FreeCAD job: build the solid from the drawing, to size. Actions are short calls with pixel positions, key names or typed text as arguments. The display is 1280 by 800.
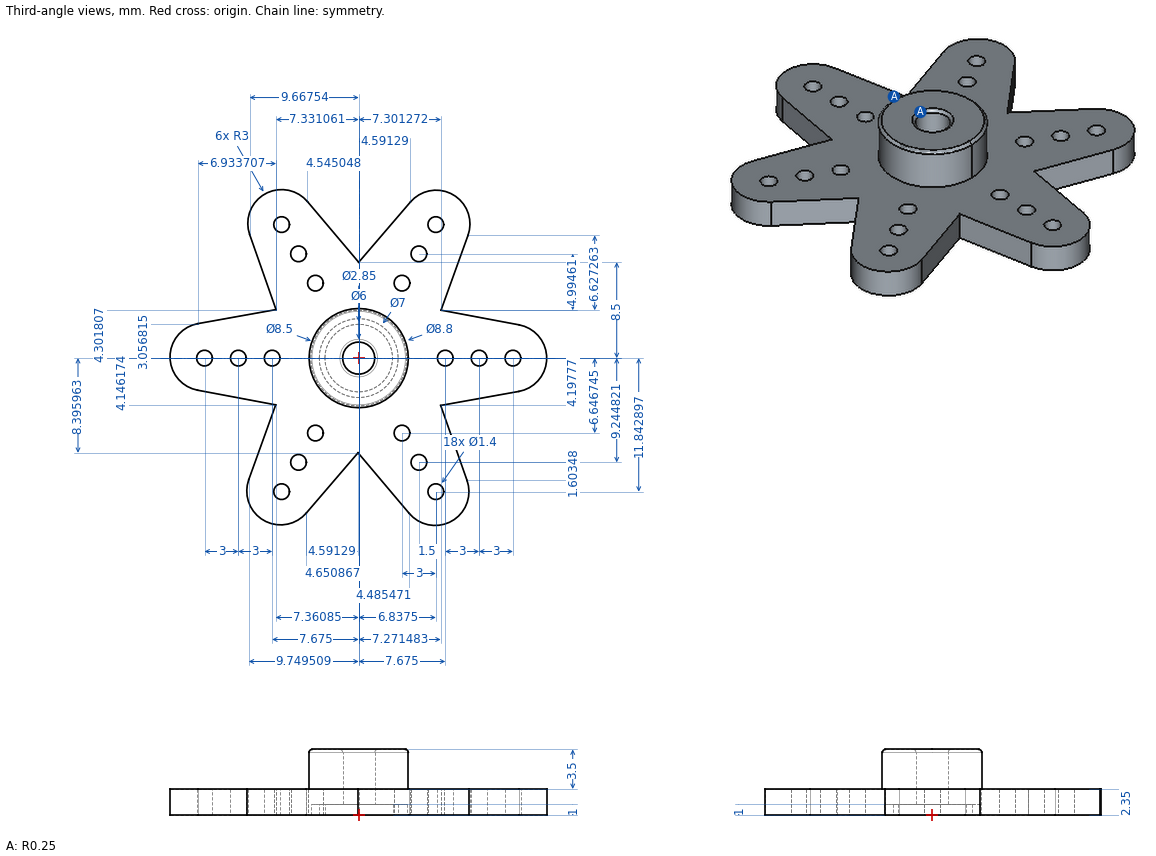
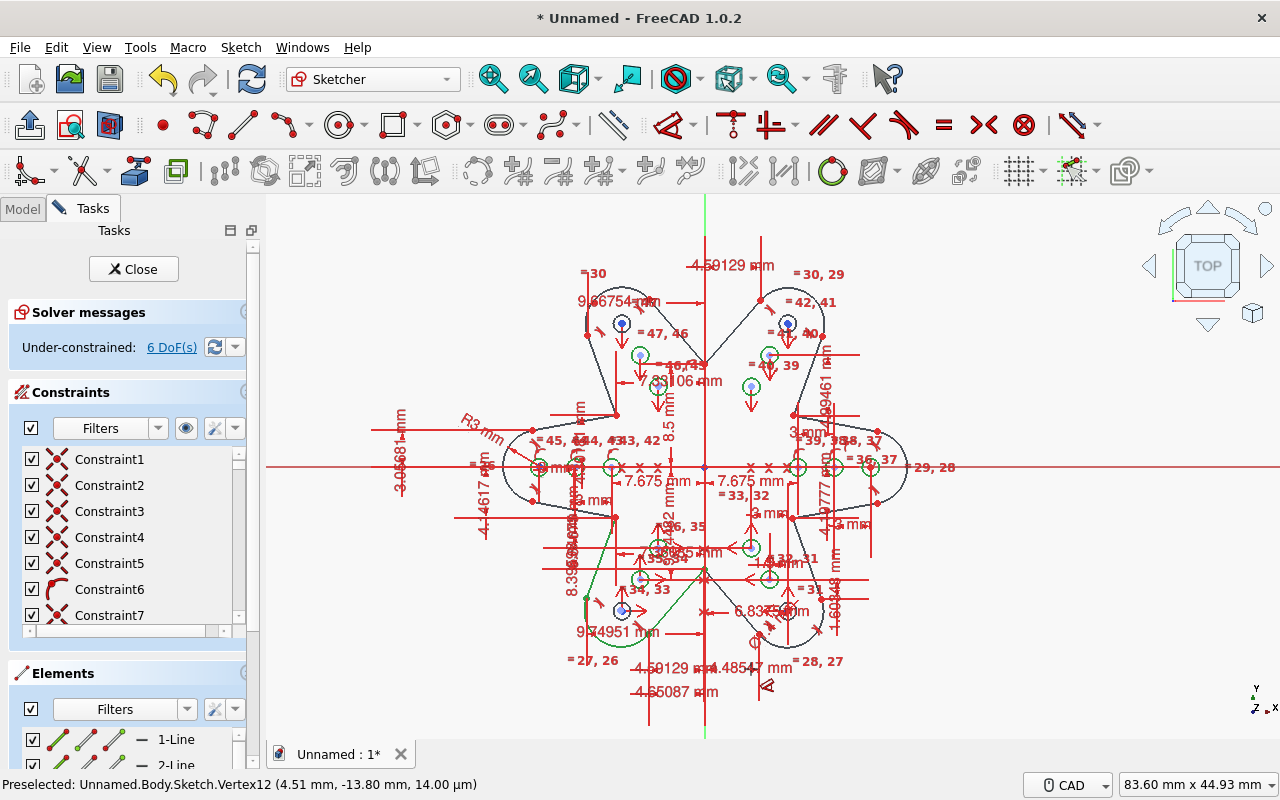
click(793, 518)
click(749, 409)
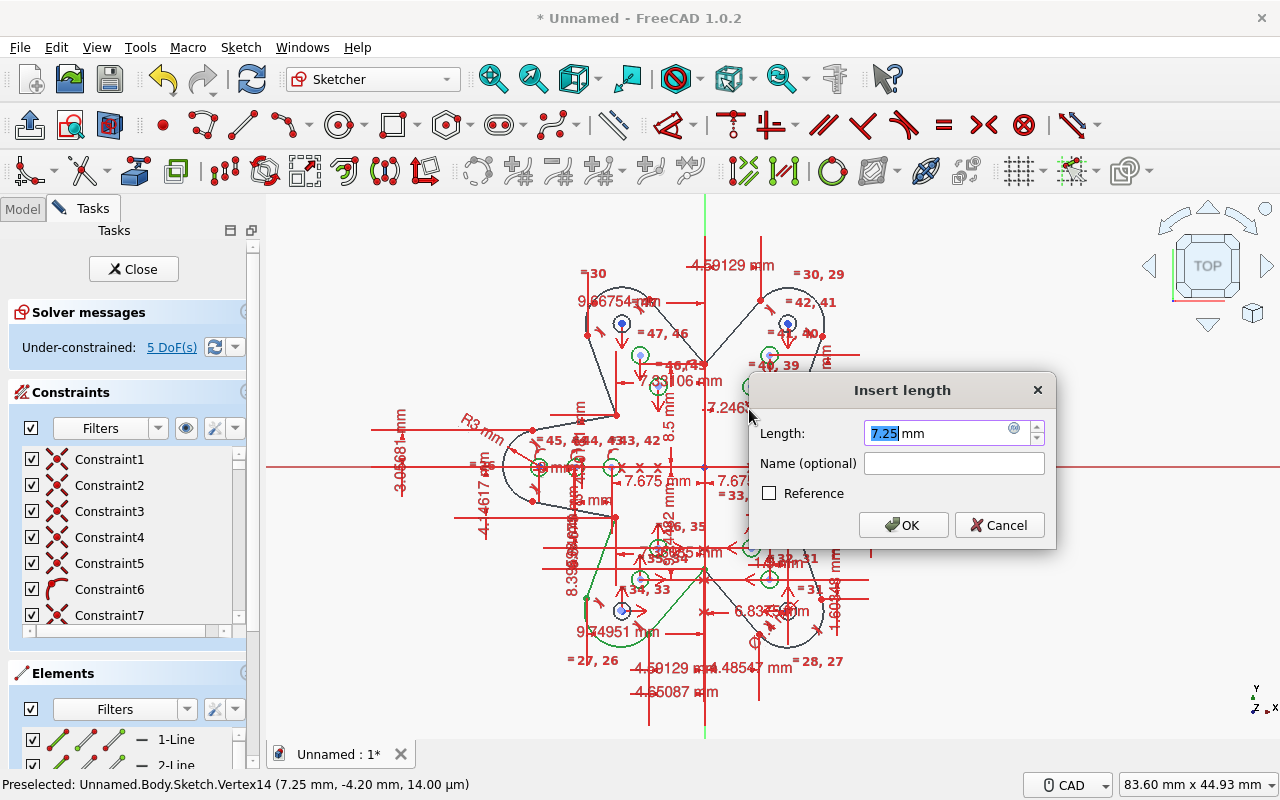
text(7.271483)
key(Return)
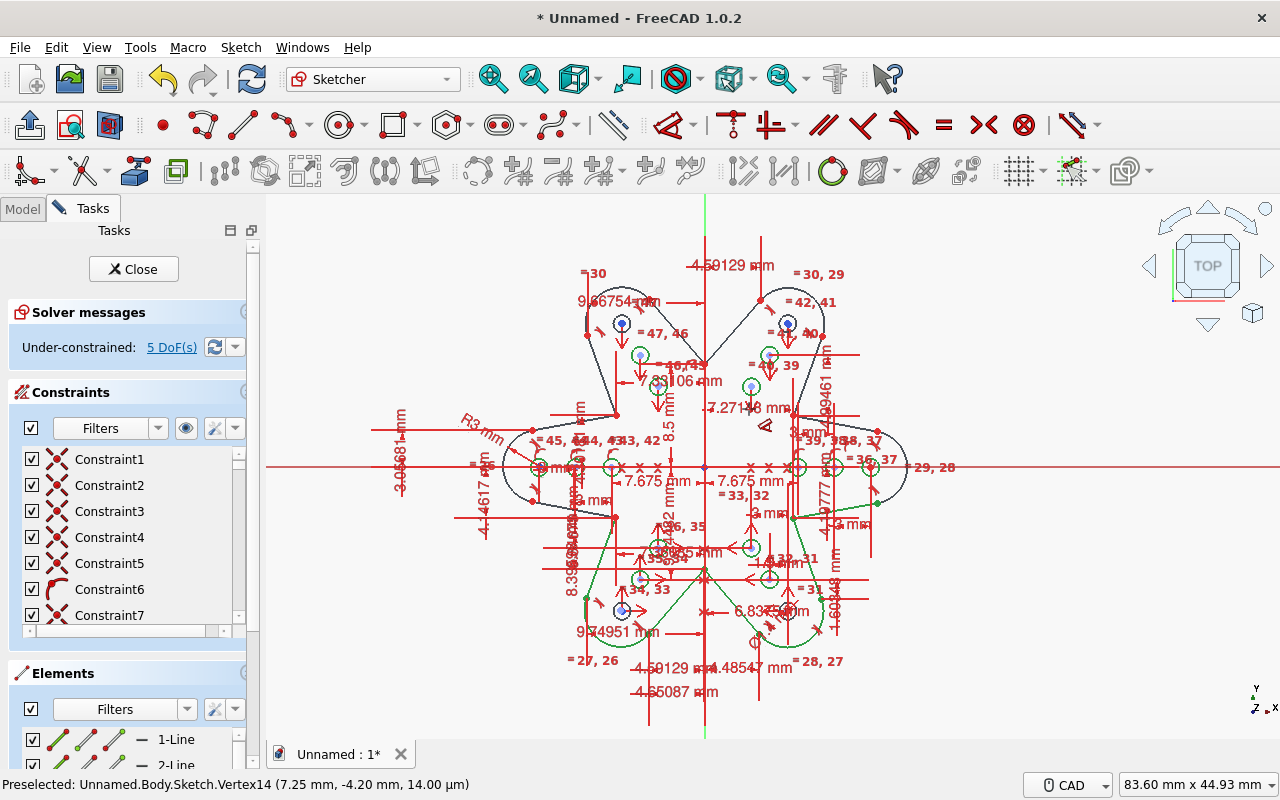
click(794, 416)
click(729, 358)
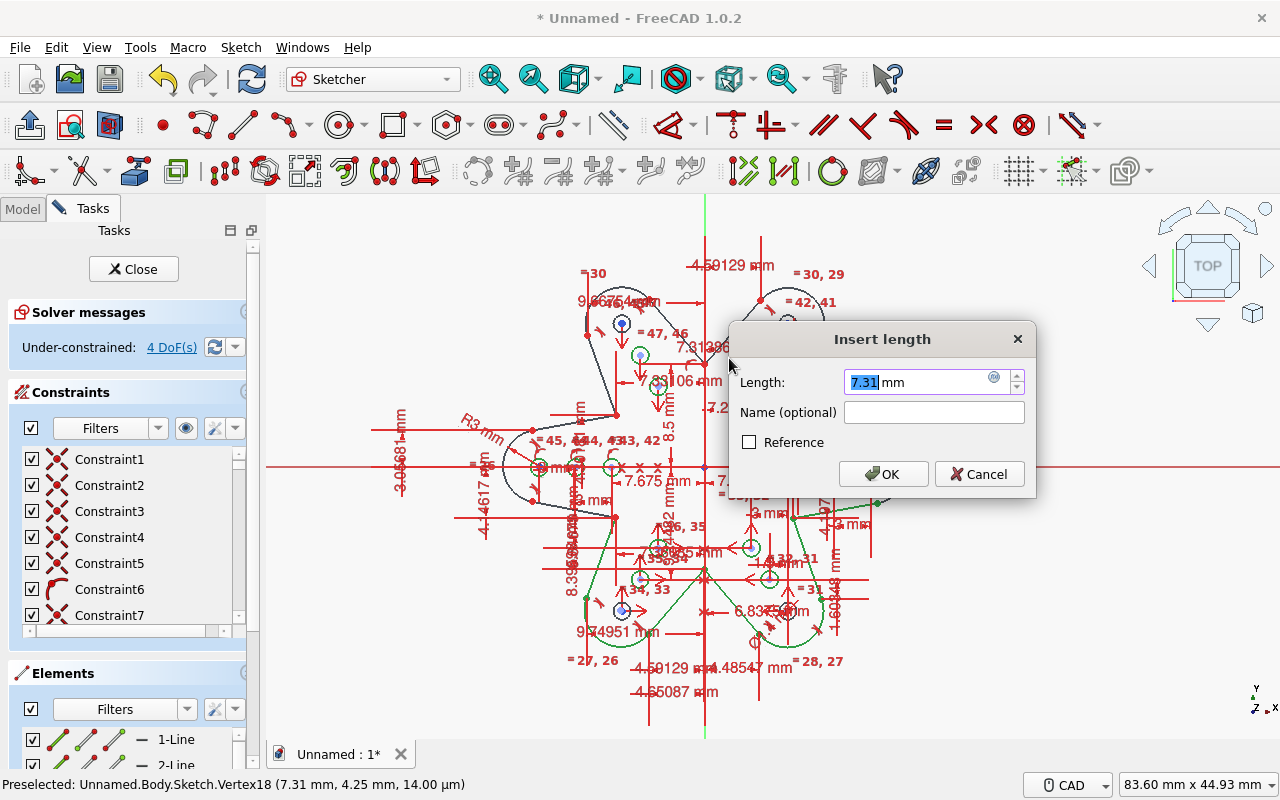
text(7.301272)
key(Return)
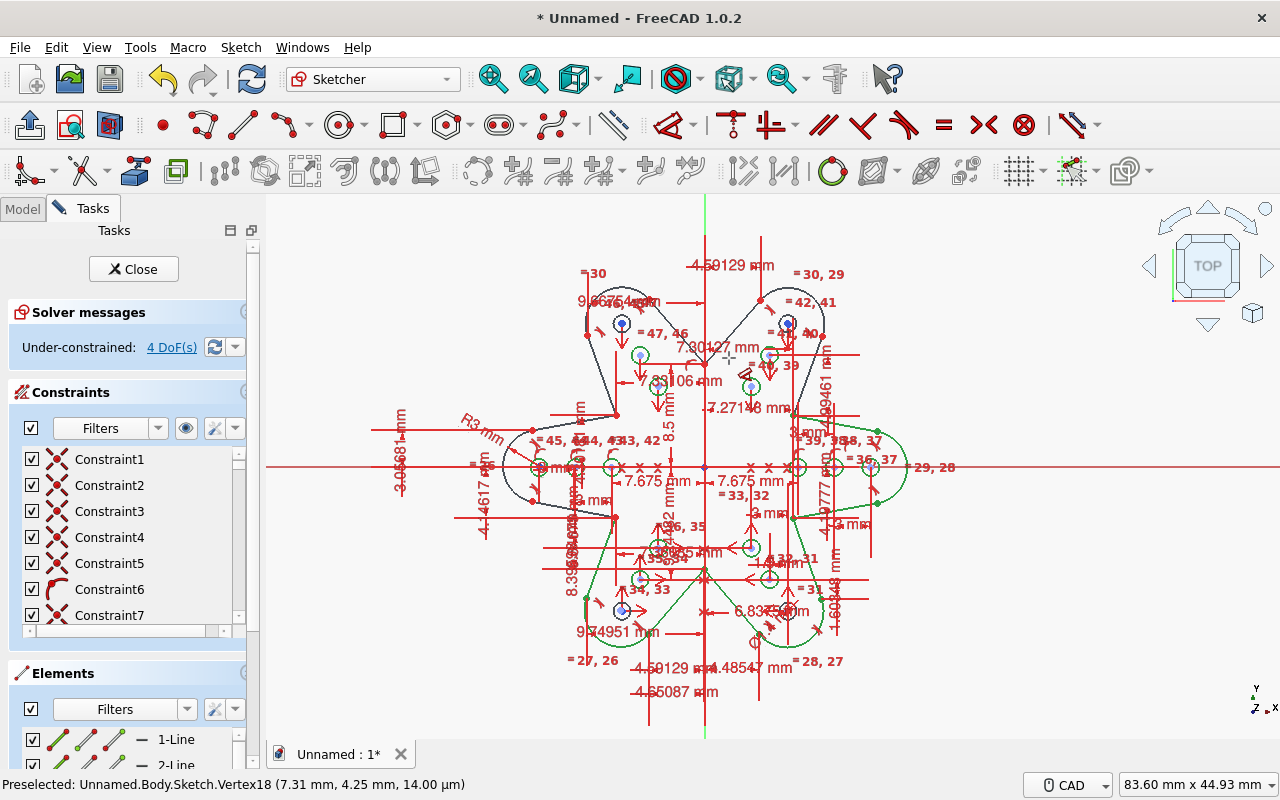
click(650, 300)
click(658, 266)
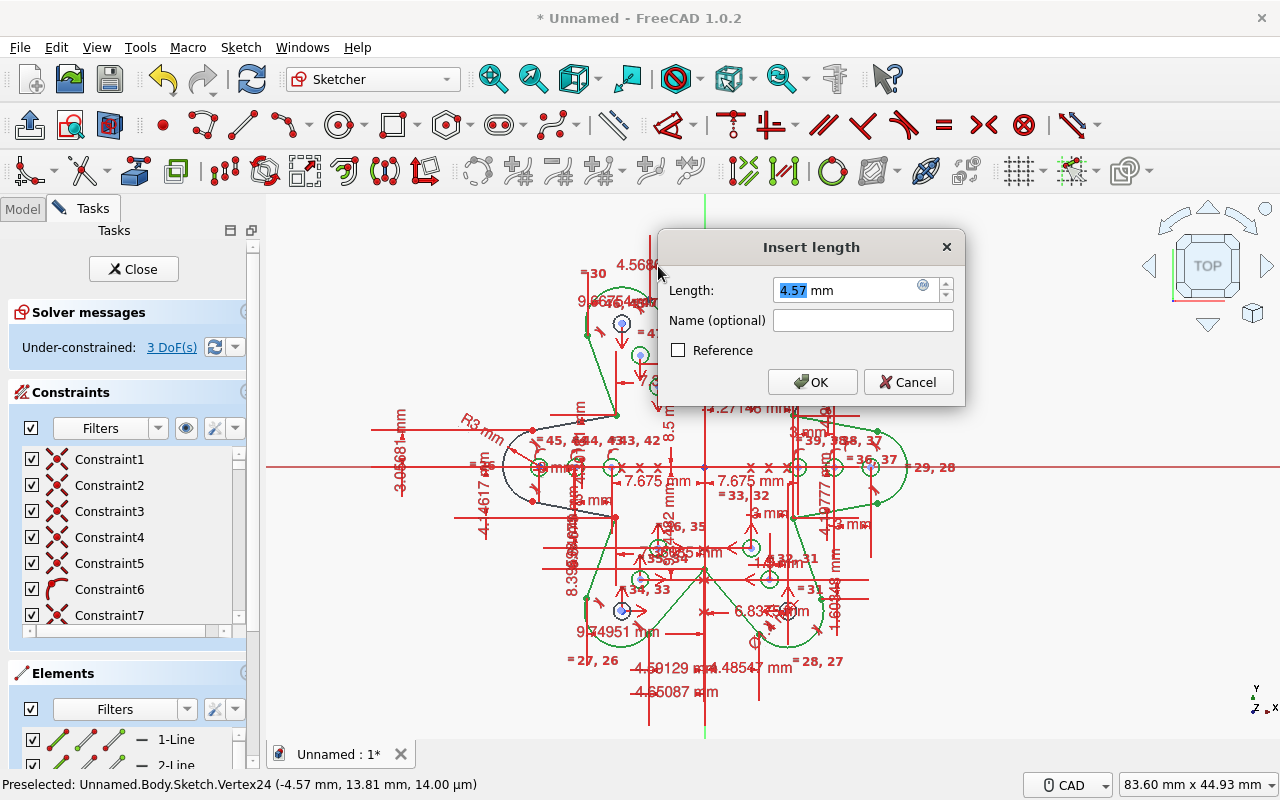
text(4.545048)
key(Return)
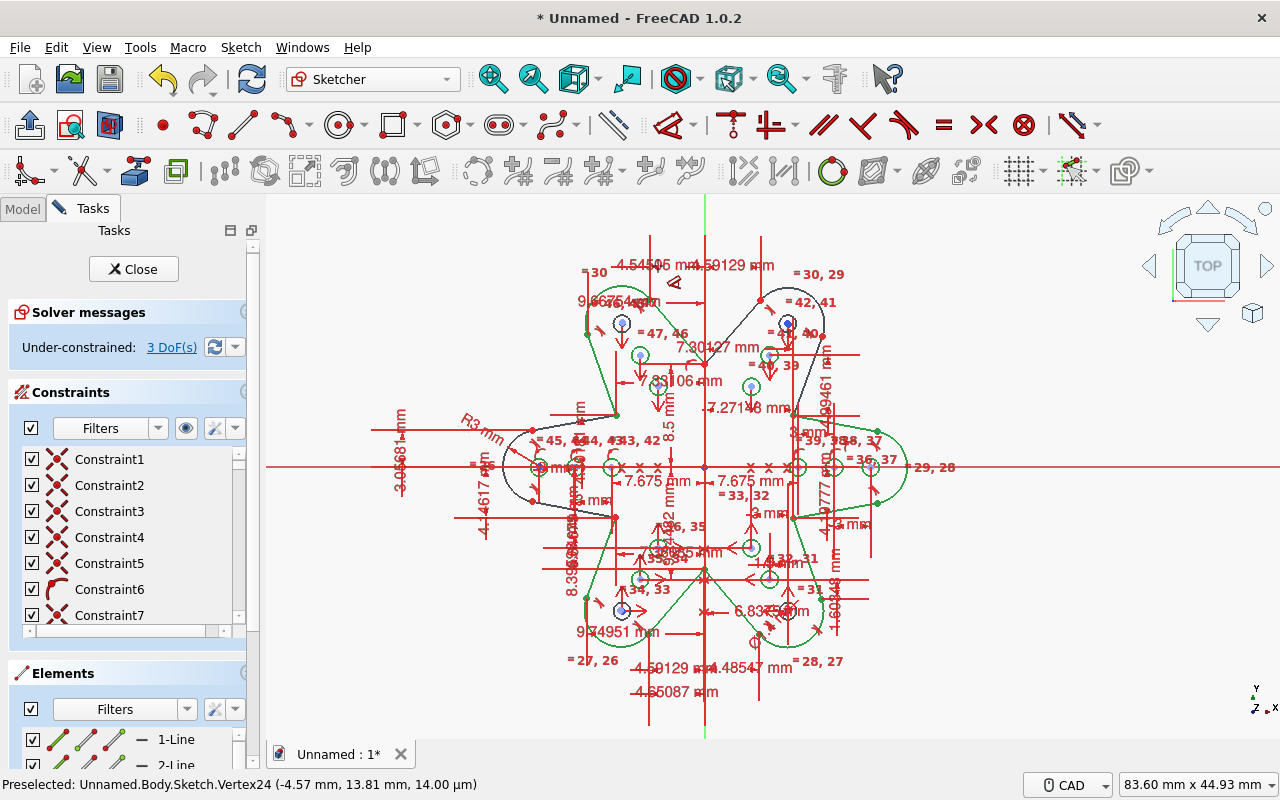
click(591, 420)
click(574, 381)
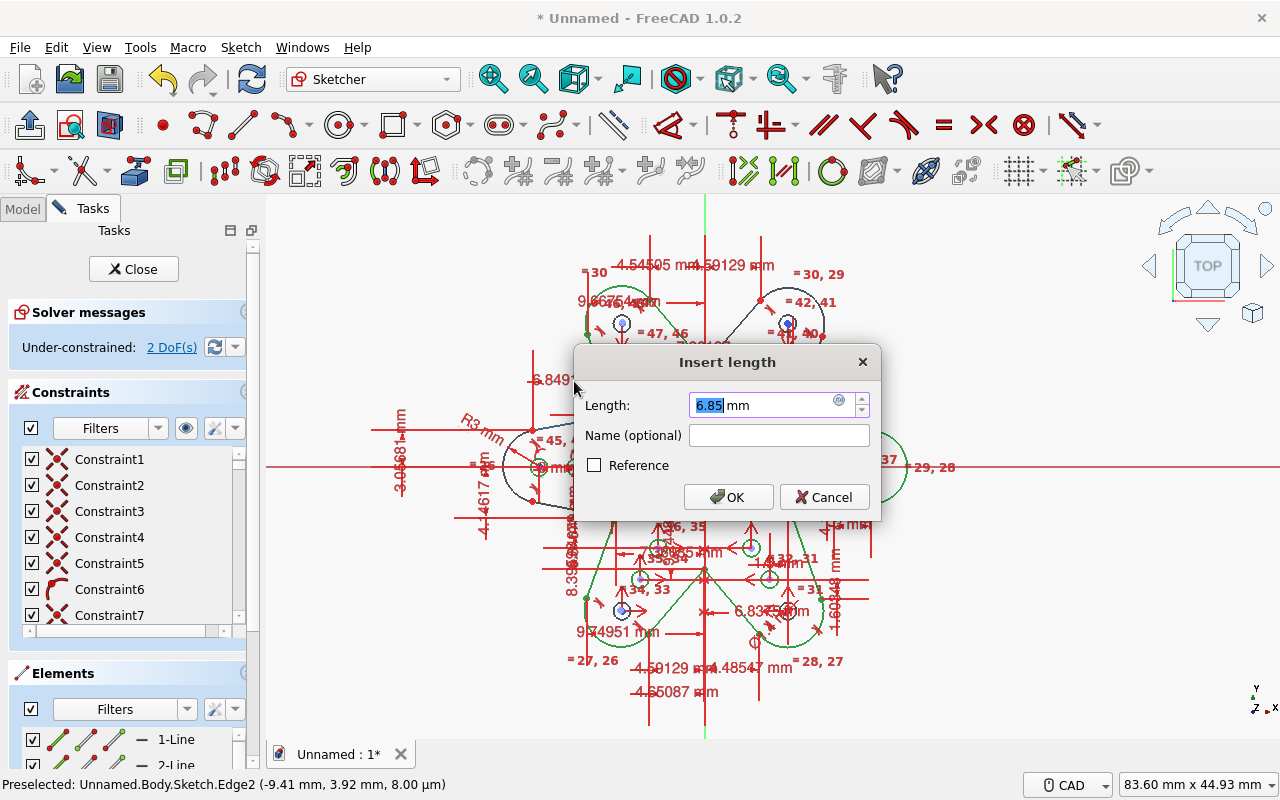
text(6.933707)
key(Return)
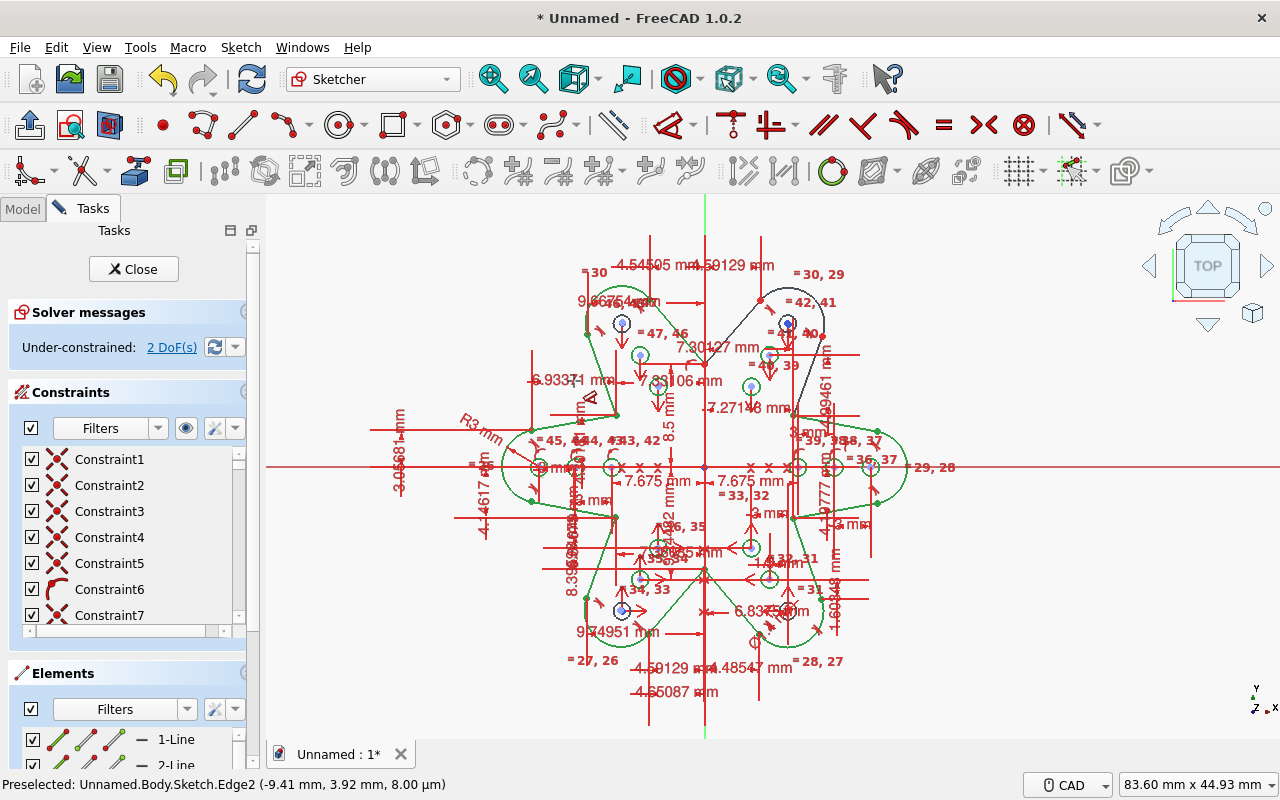
click(802, 392)
click(856, 358)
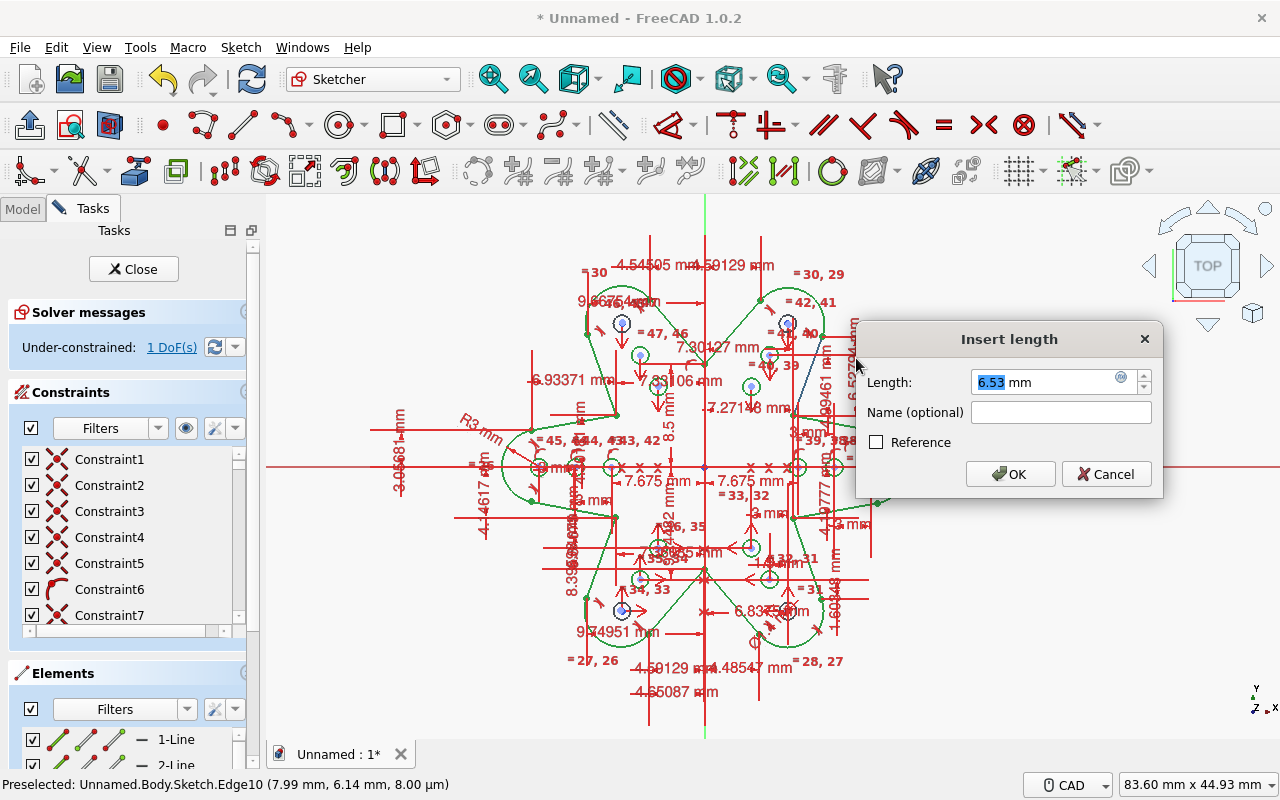
text(6.627263)
key(Return)